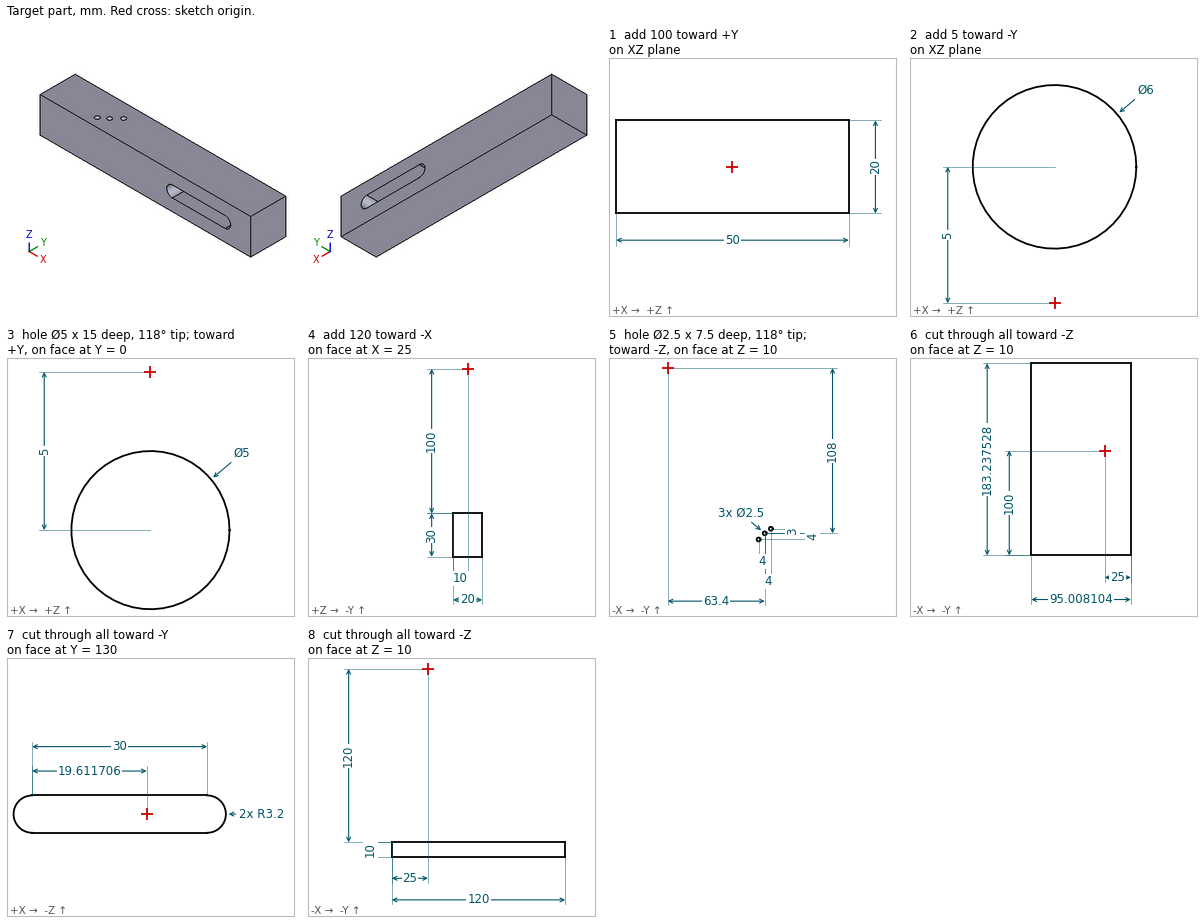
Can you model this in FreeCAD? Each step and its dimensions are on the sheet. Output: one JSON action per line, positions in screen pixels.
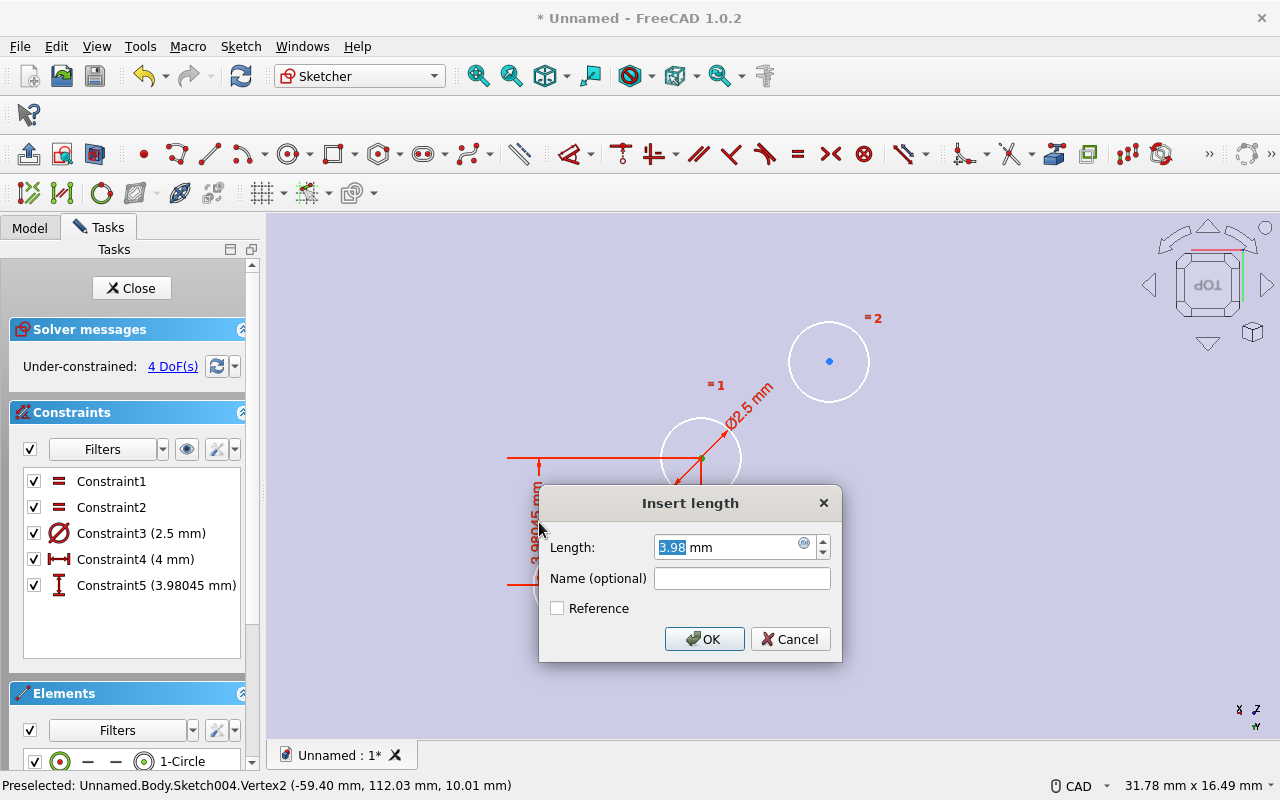
{"action": "type", "text": "4"}
{"action": "key", "text": "Return"}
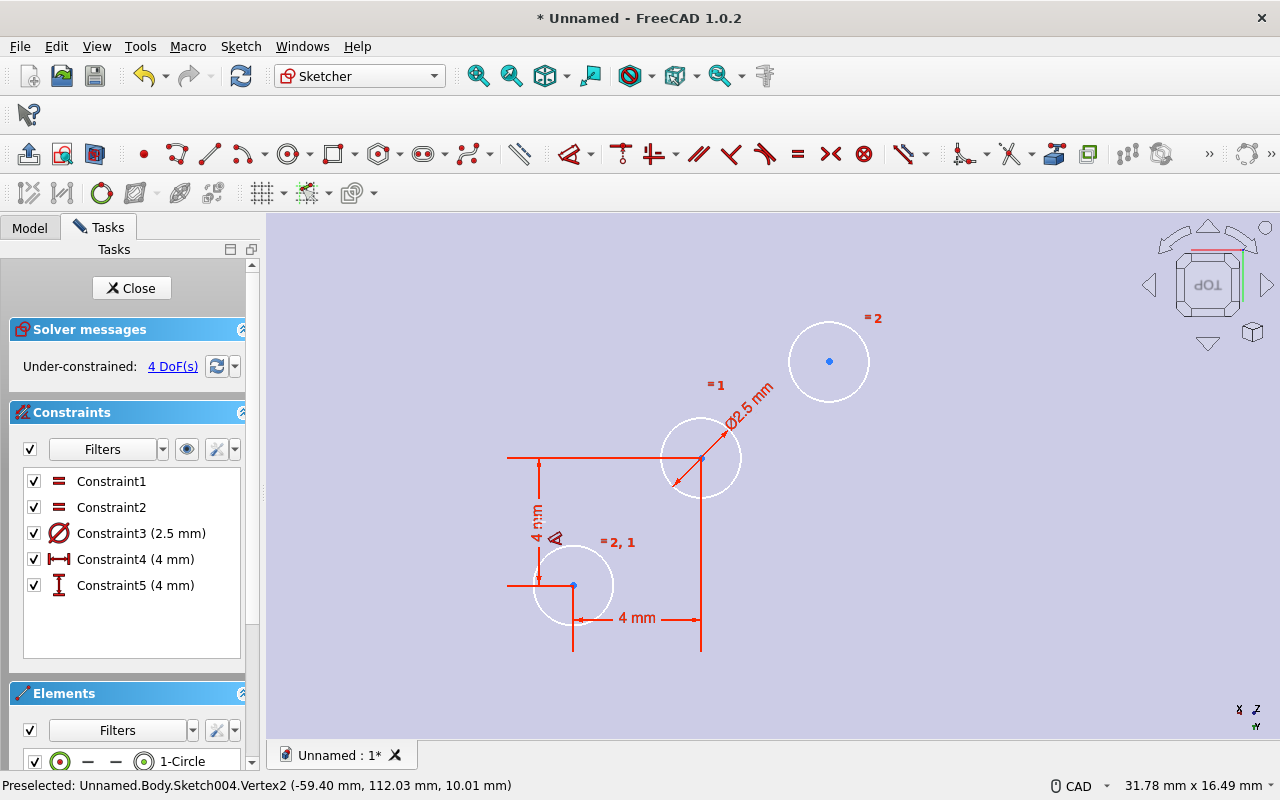
{"action": "left_click", "coordinate": [701, 458]}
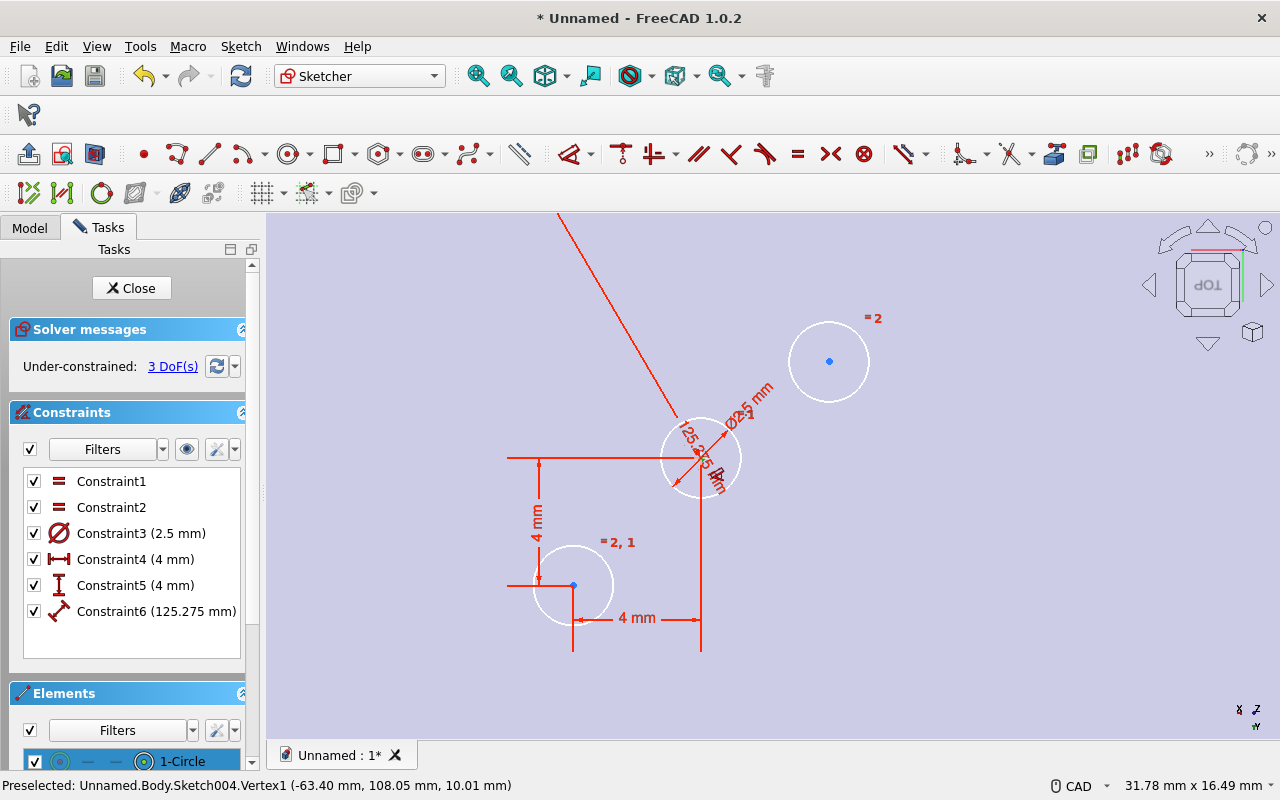
{"action": "left_click", "coordinate": [829, 362]}
{"action": "left_click", "coordinate": [765, 328]}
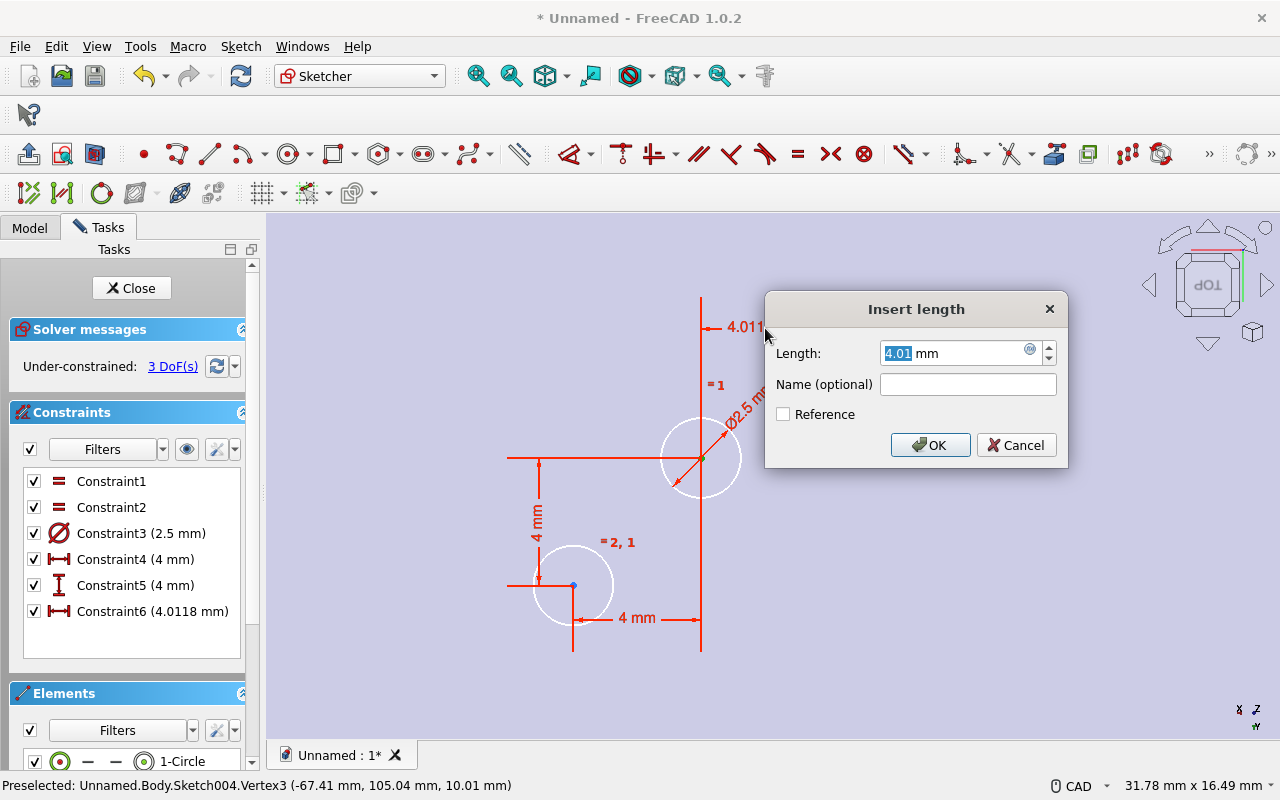
{"action": "type", "text": "4"}
{"action": "key", "text": "Return"}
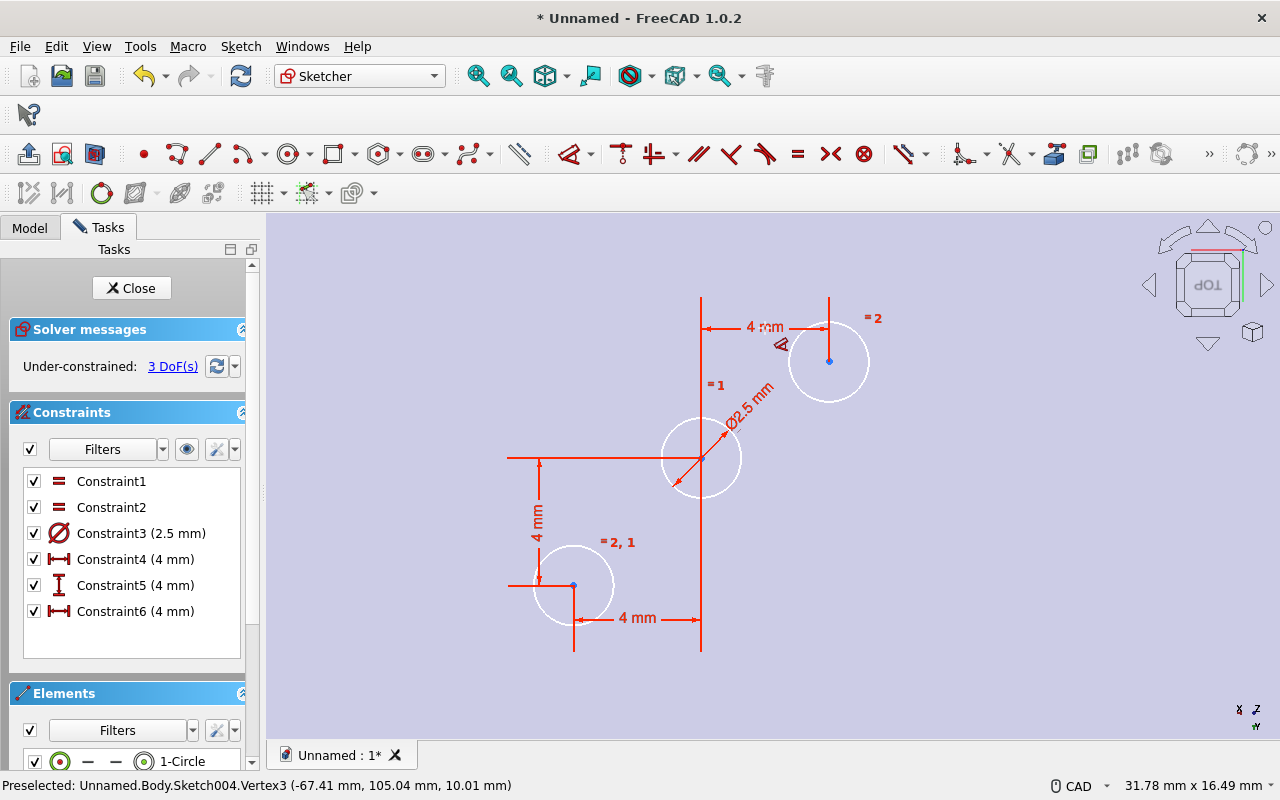
{"action": "left_click", "coordinate": [701, 458]}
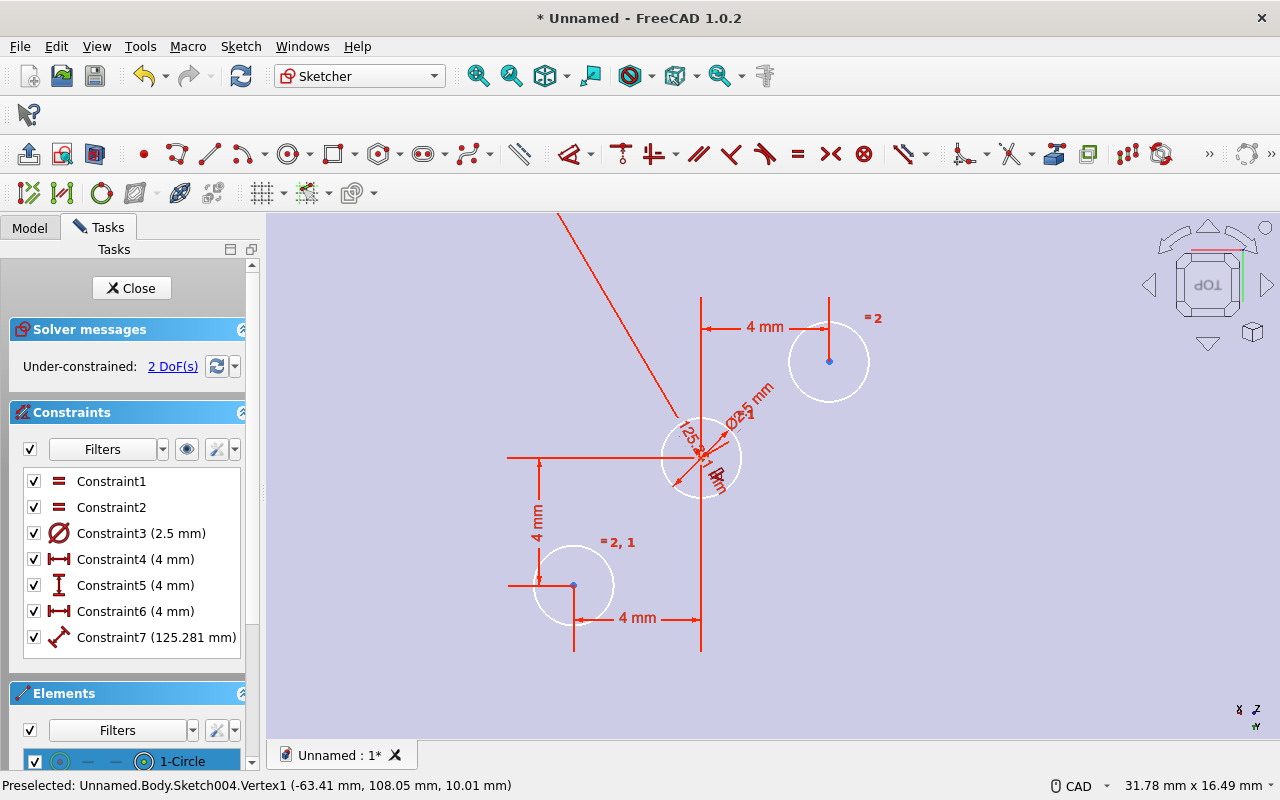
{"action": "left_click", "coordinate": [829, 362]}
{"action": "left_click", "coordinate": [863, 410]}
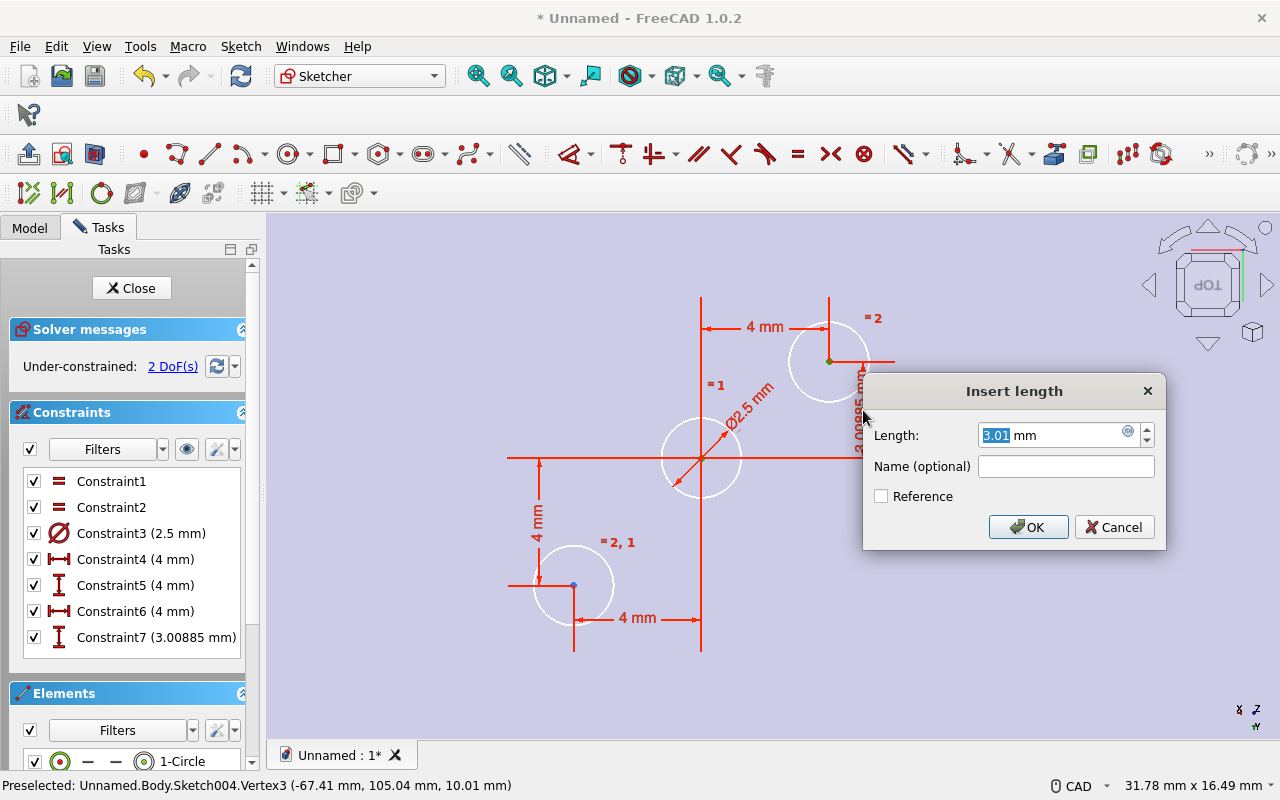
{"action": "type", "text": "3"}
{"action": "key", "text": "Return"}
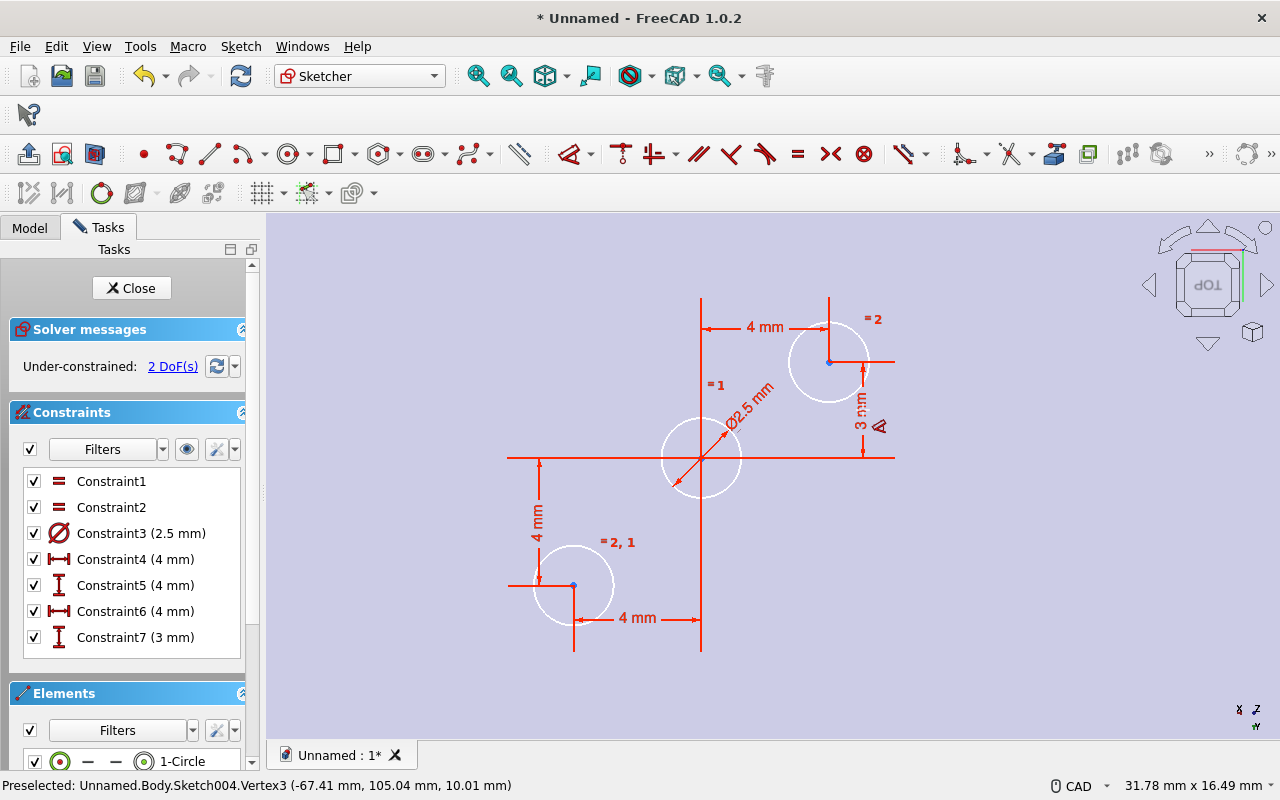
{"action": "left_click", "coordinate": [701, 458]}
{"action": "left_click", "coordinate": [735, 350]}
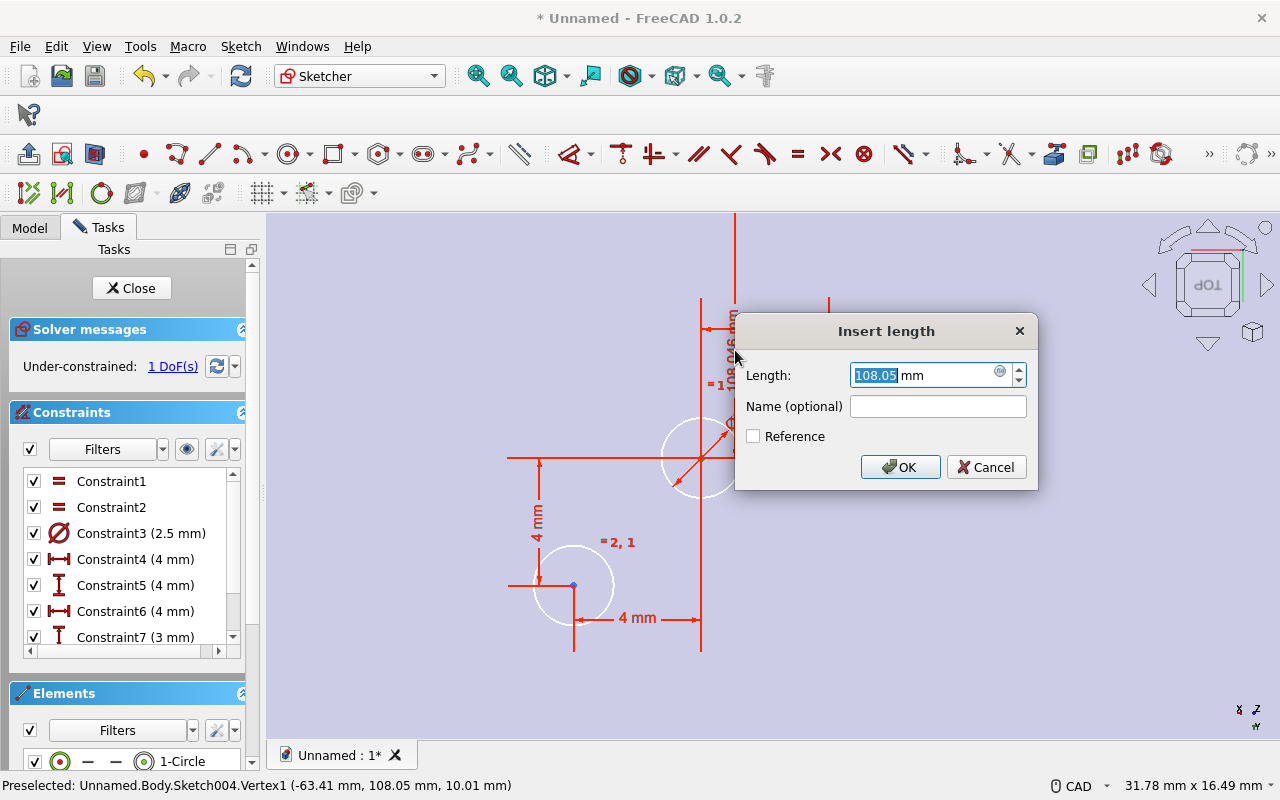
{"action": "type", "text": "108"}
{"action": "key", "text": "Return"}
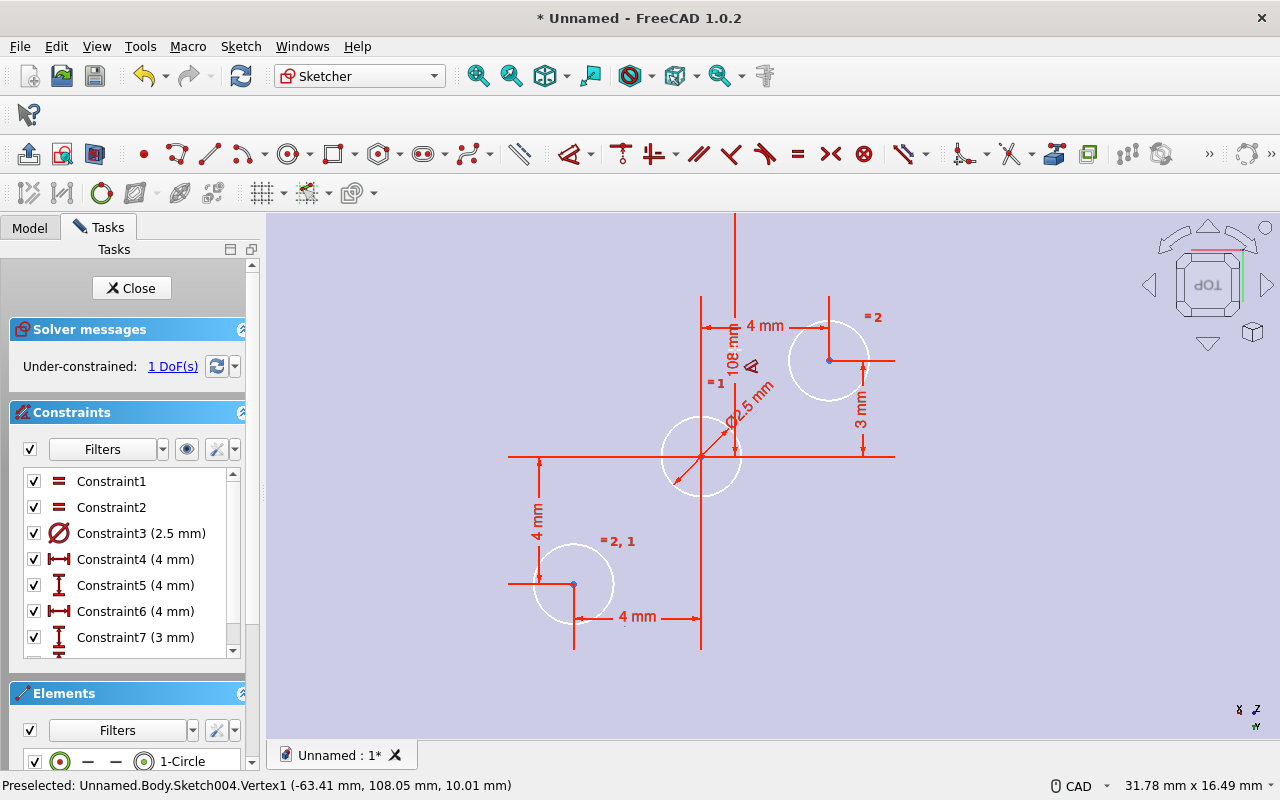
{"action": "left_click", "coordinate": [701, 457]}
{"action": "left_click", "coordinate": [498, 491]}